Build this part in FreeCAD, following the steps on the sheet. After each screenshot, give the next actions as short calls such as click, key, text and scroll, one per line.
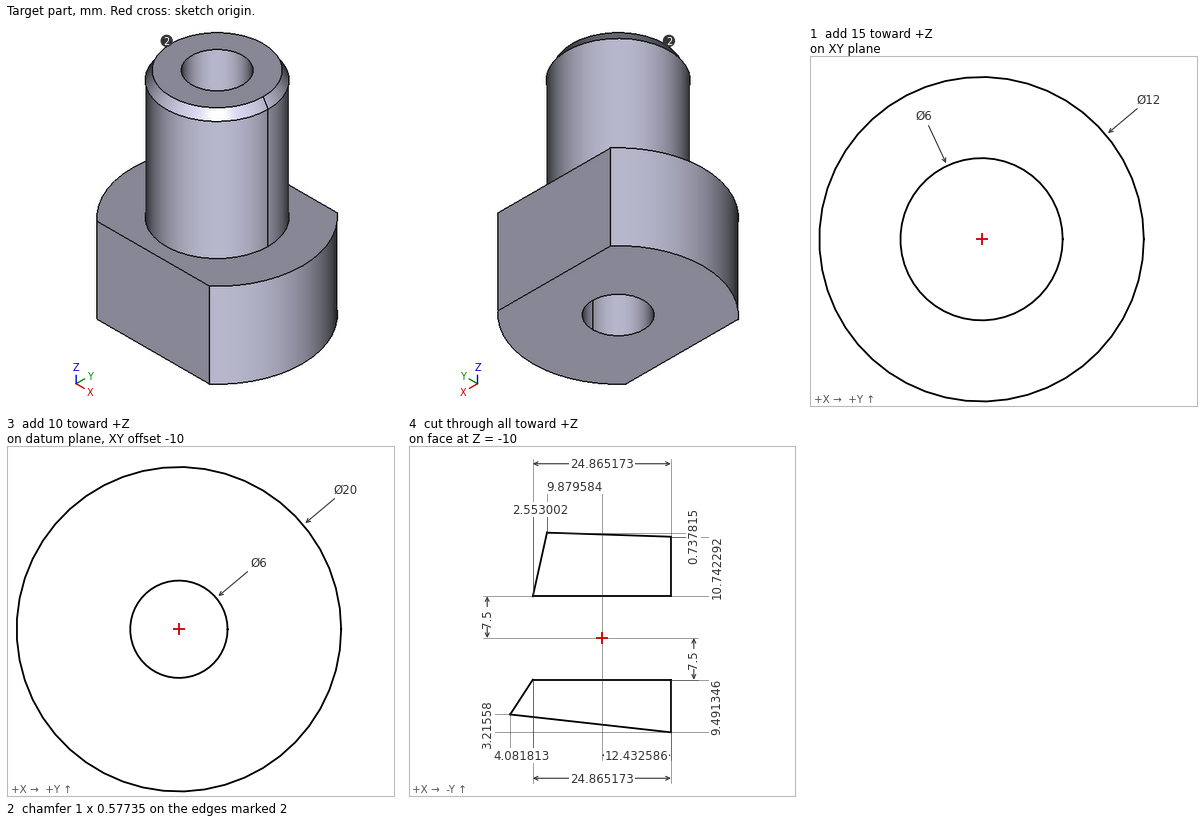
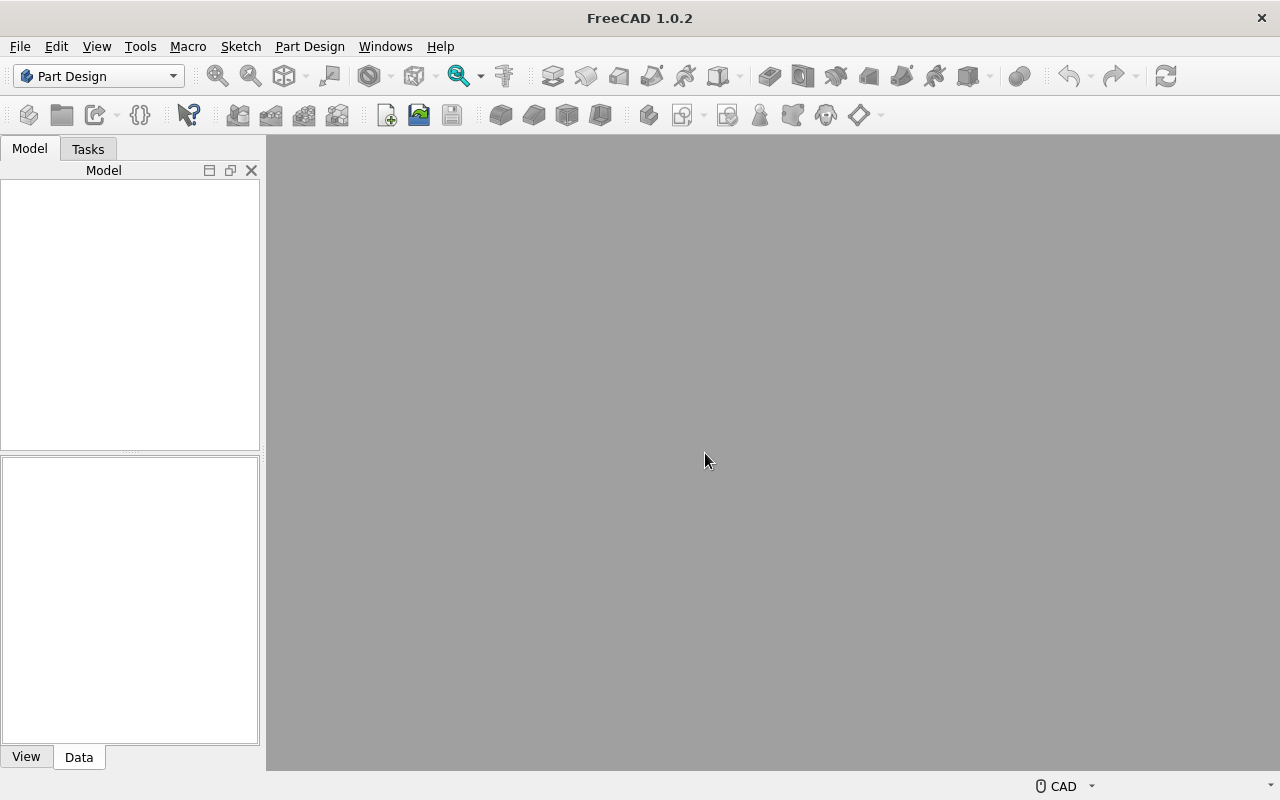
click(386, 116)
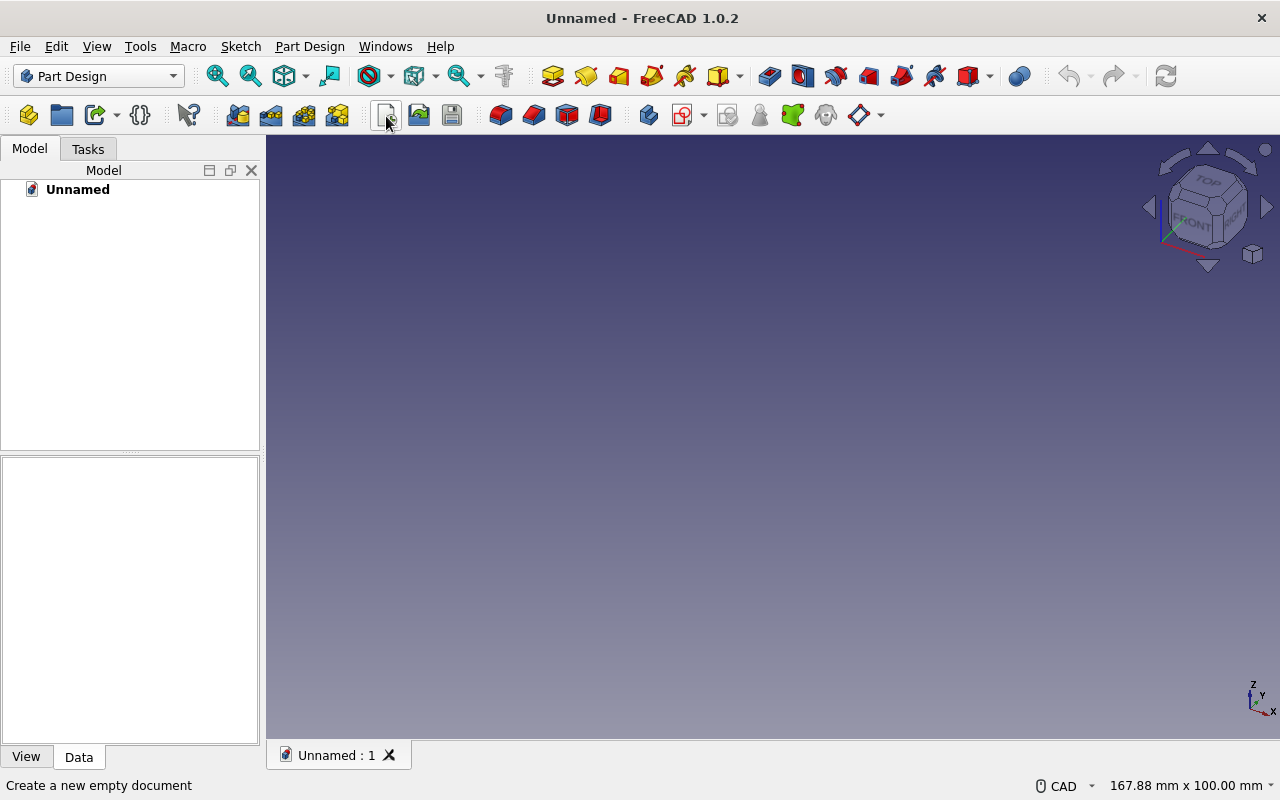
click(682, 116)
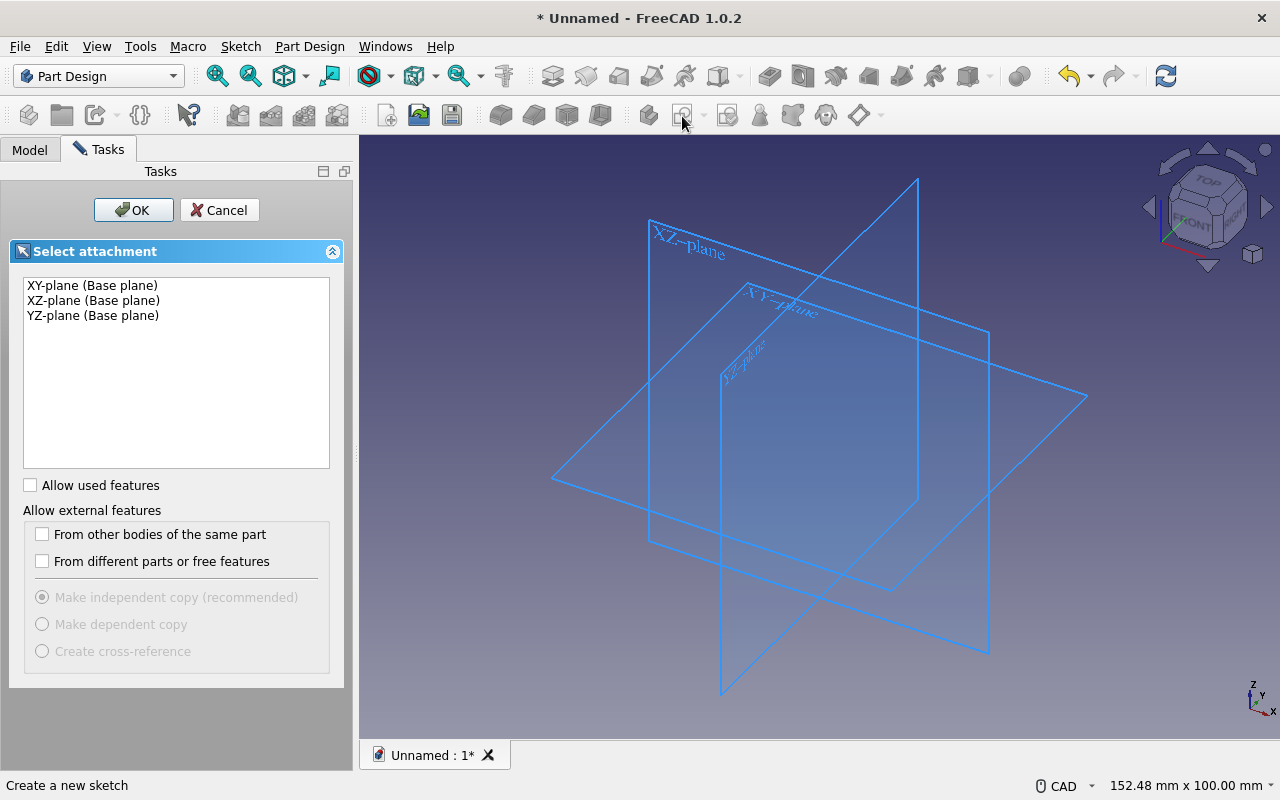
click(84, 286)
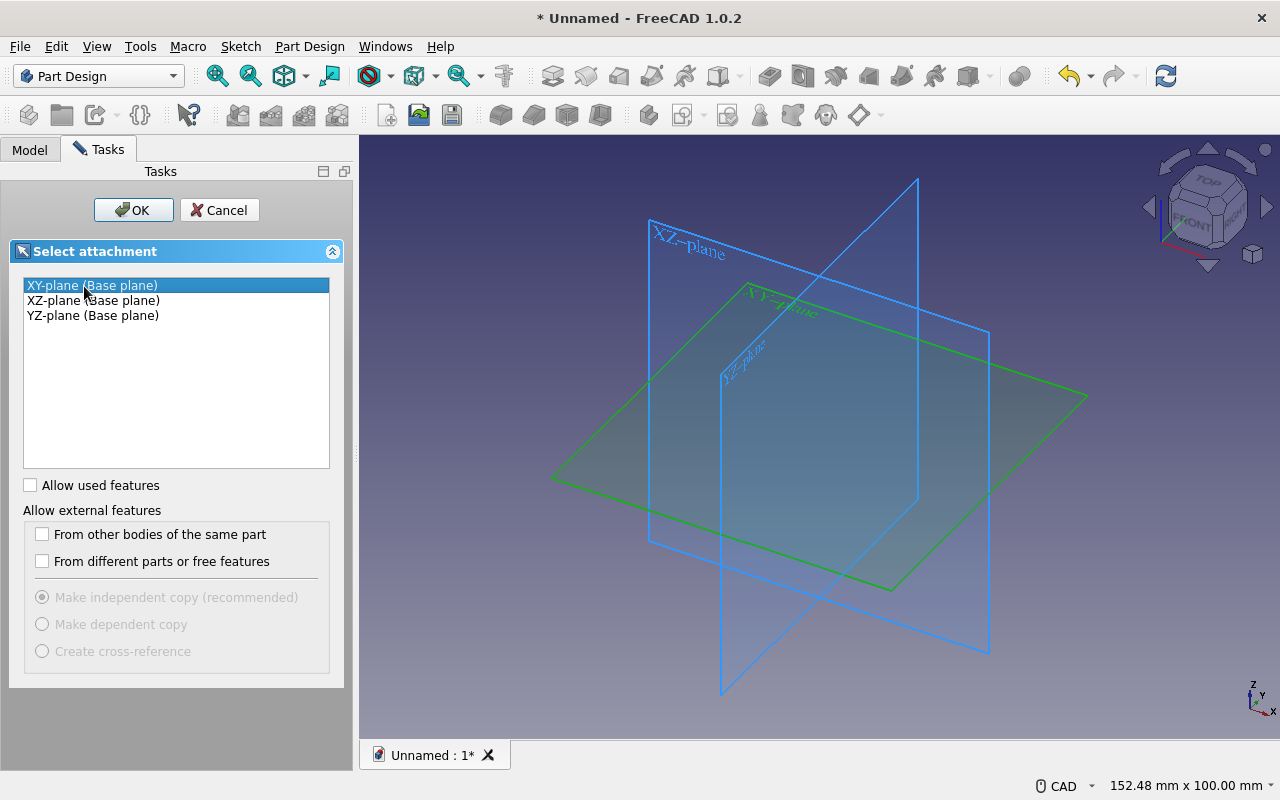
click(134, 210)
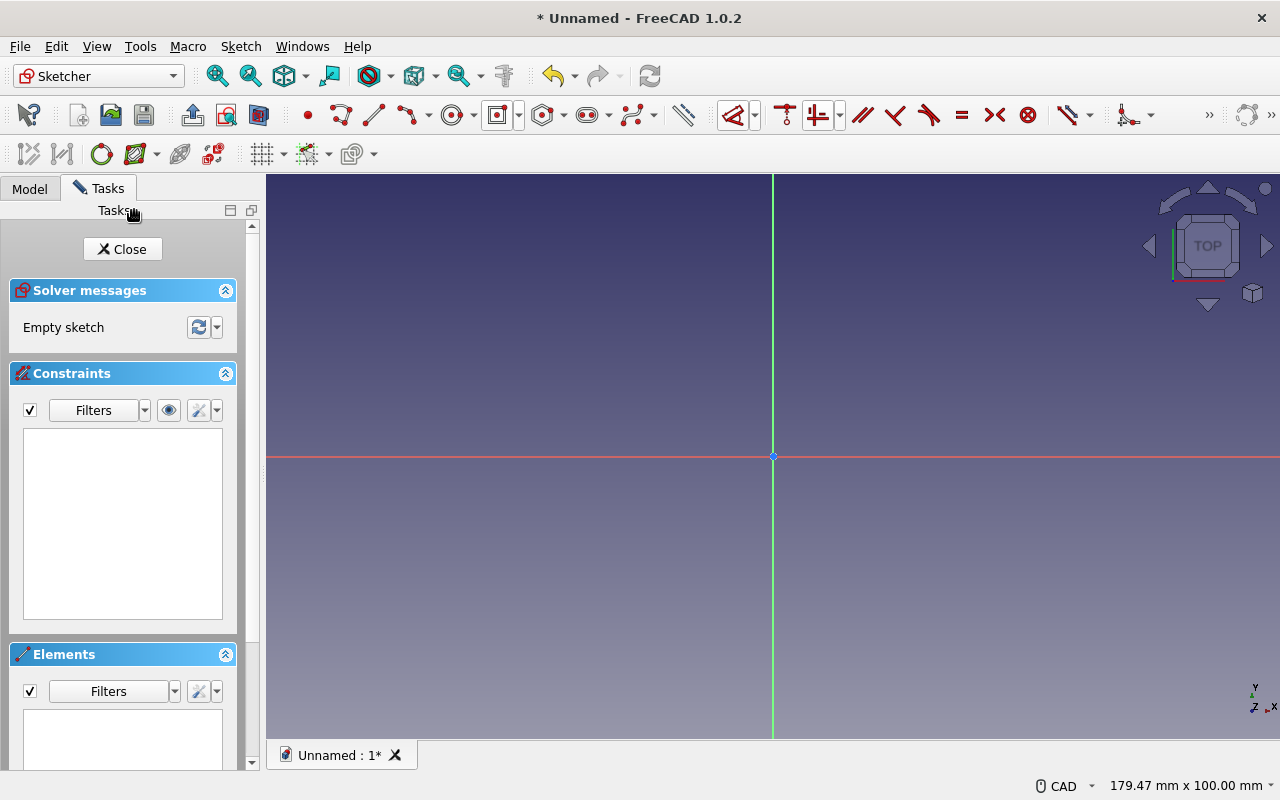
scroll(790, 456, up, 8)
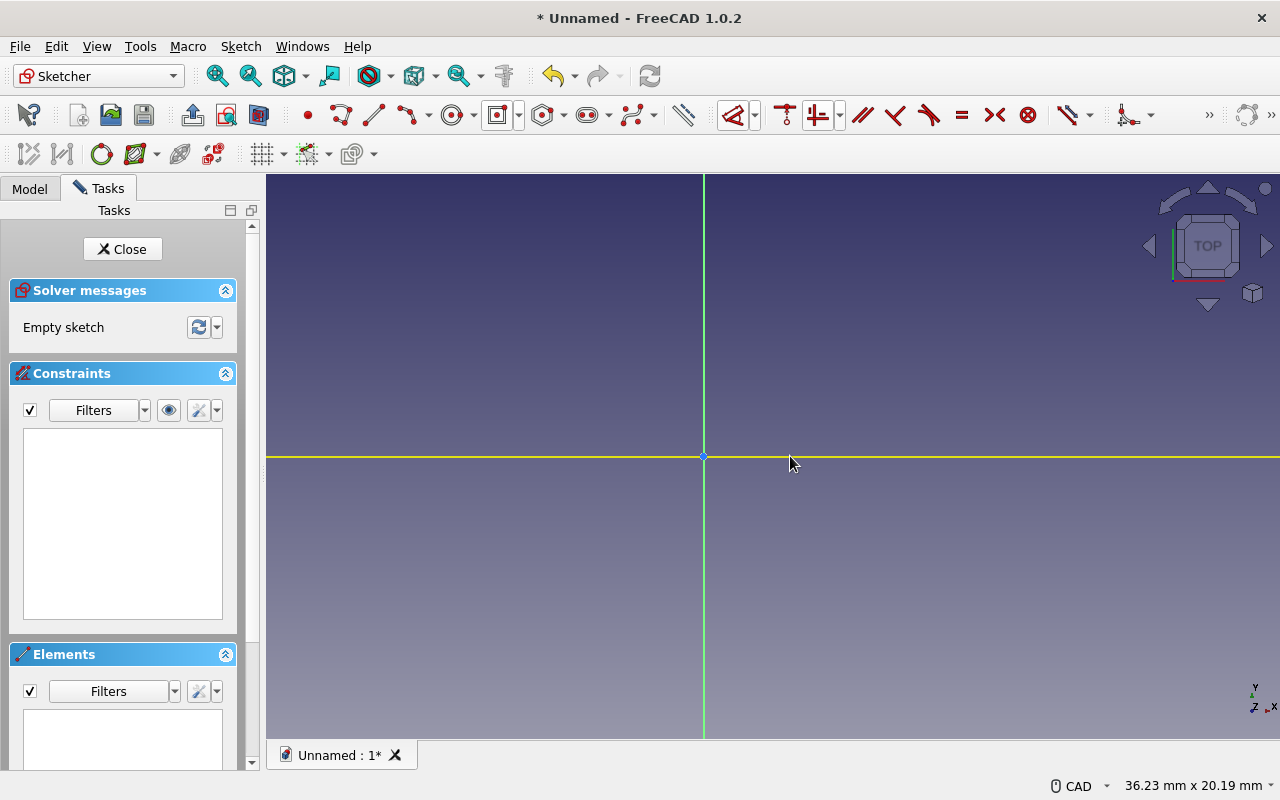
click(452, 116)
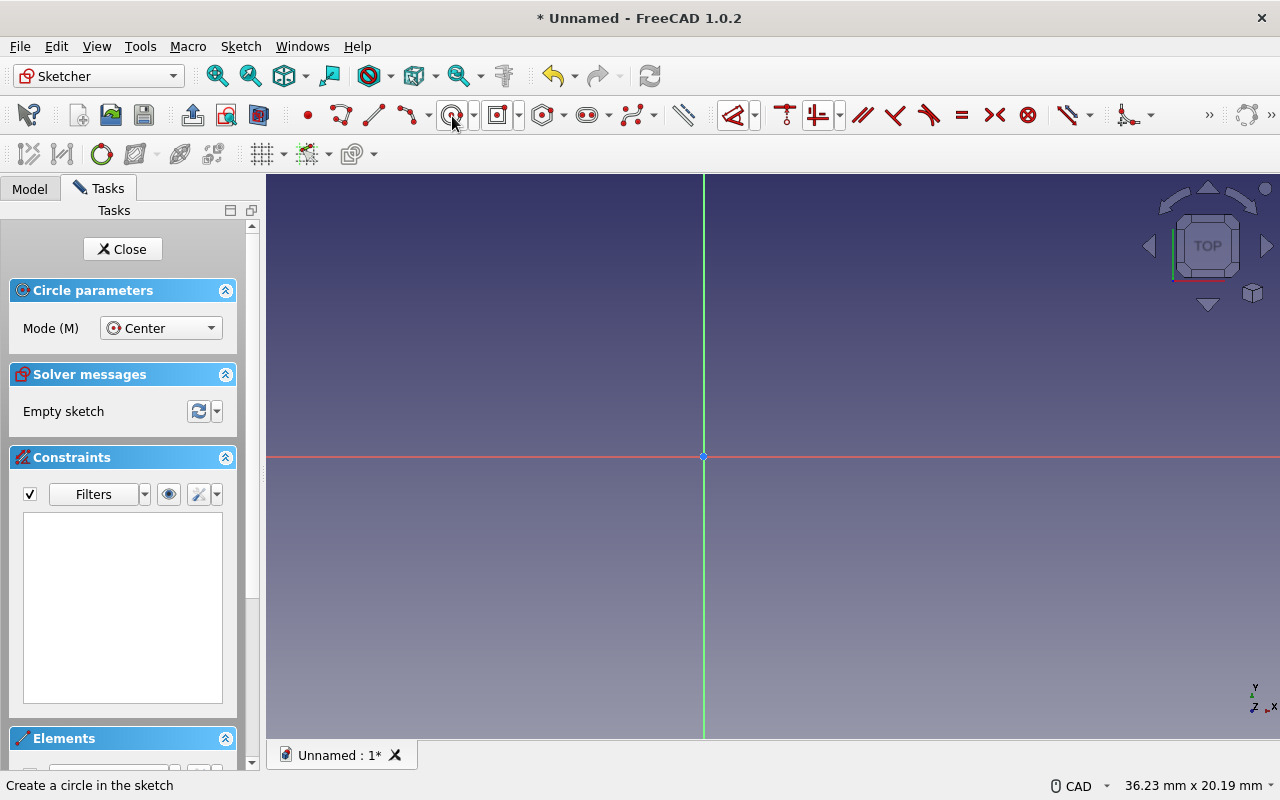
click(704, 456)
move(822, 338)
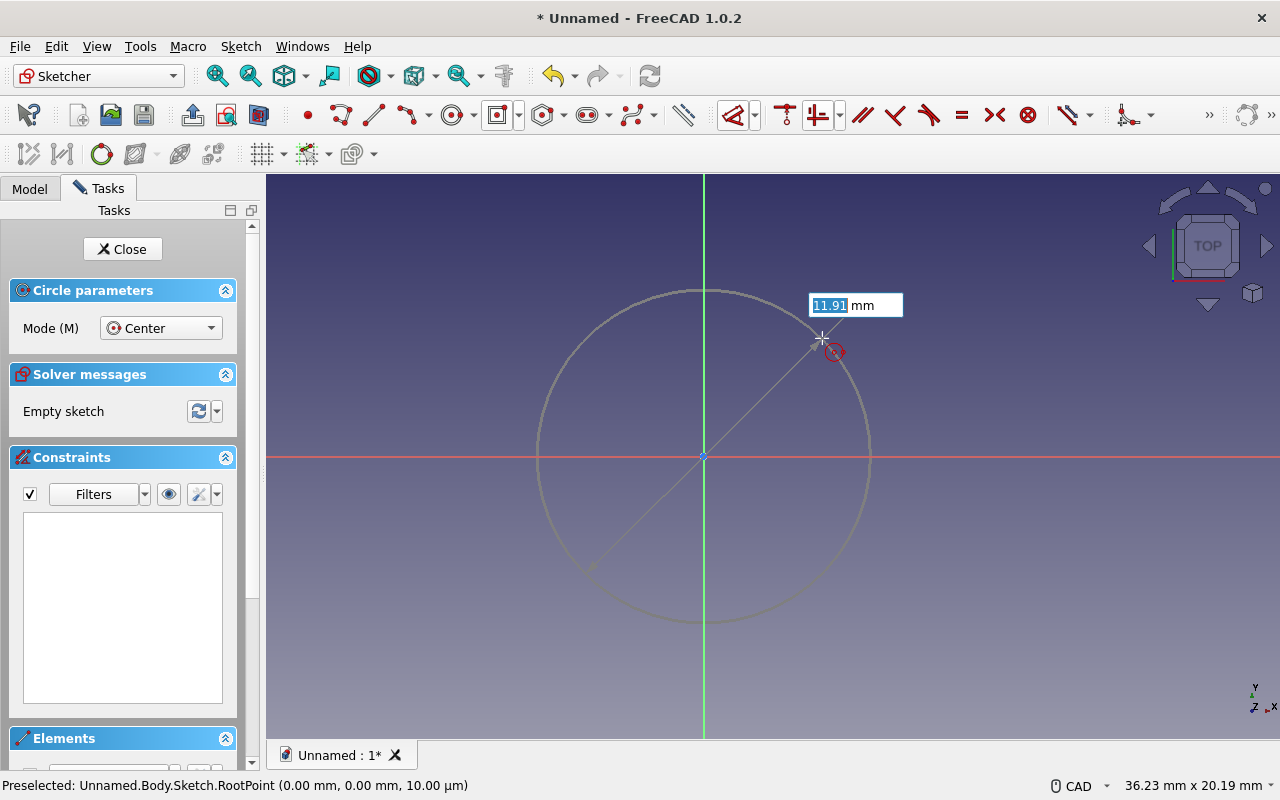
text(12)
key(Return)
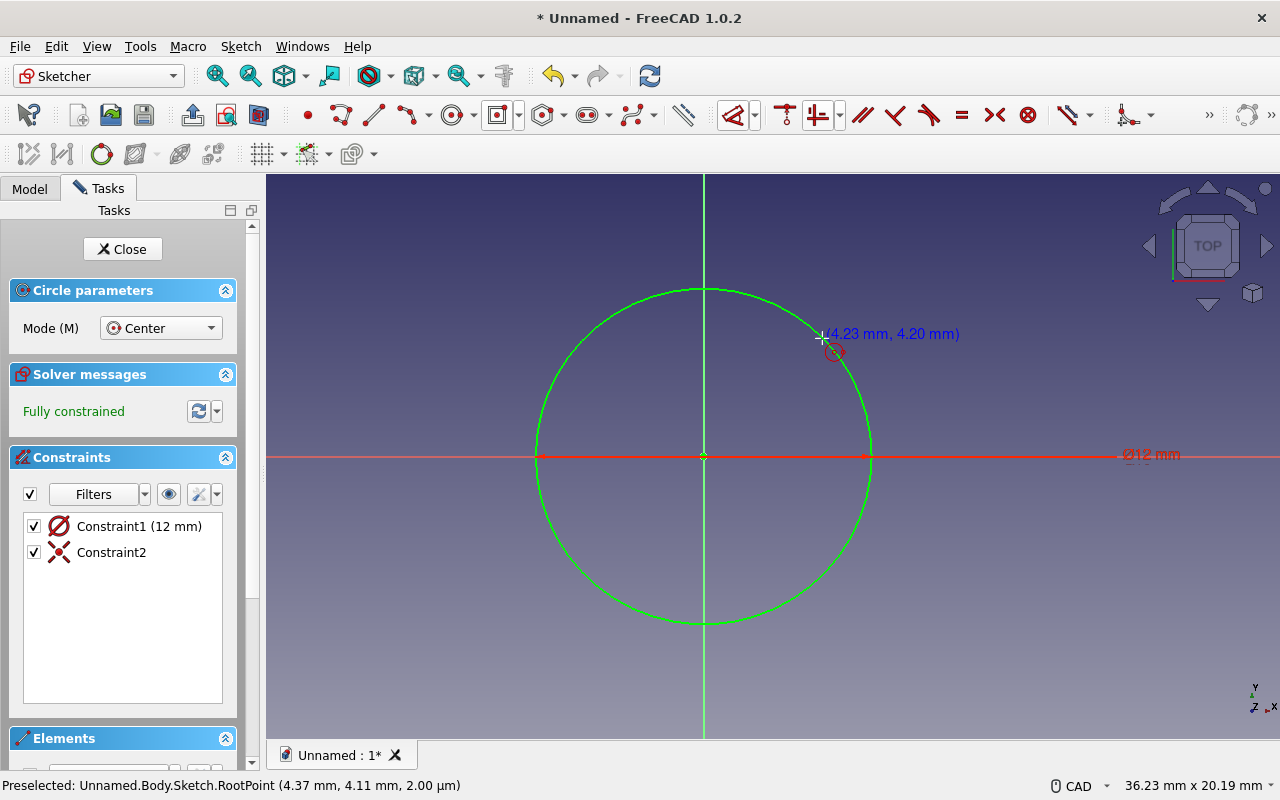
click(704, 456)
move(763, 397)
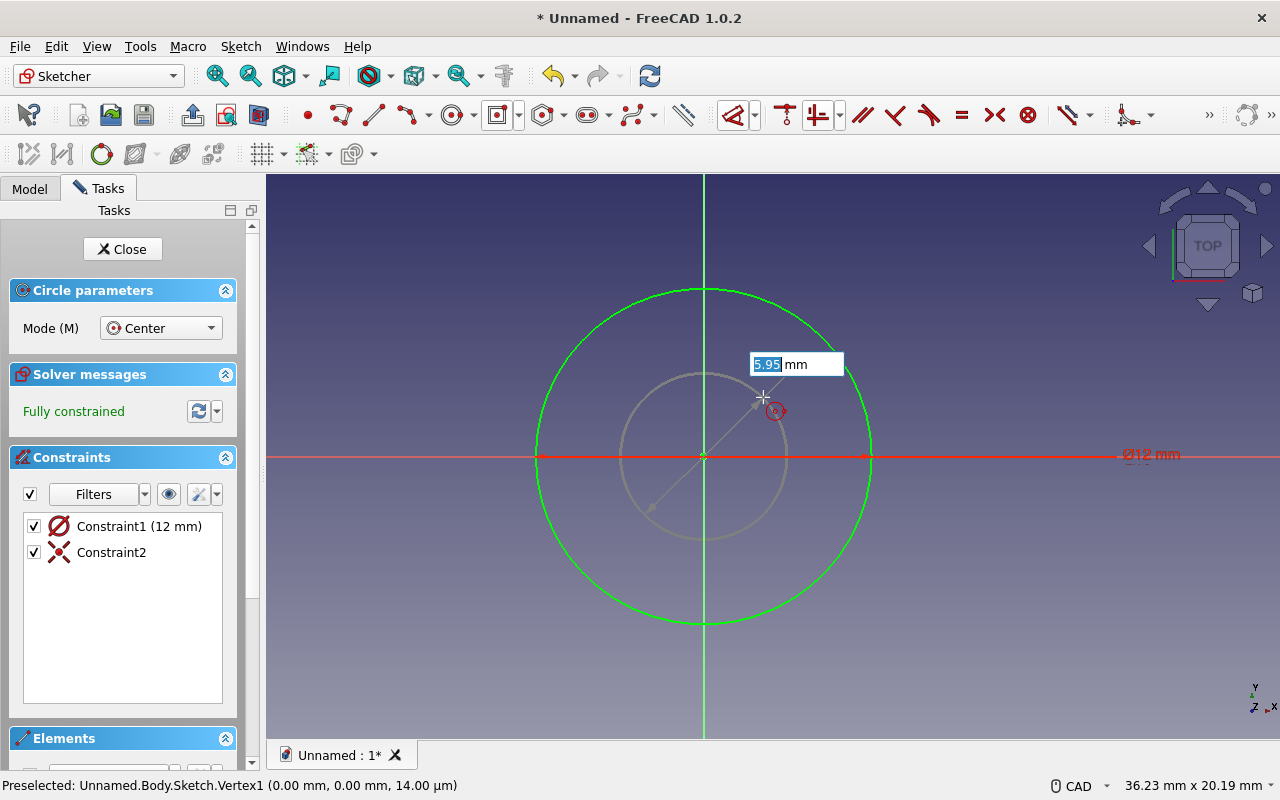
text(6)
key(Return)
key(Escape)